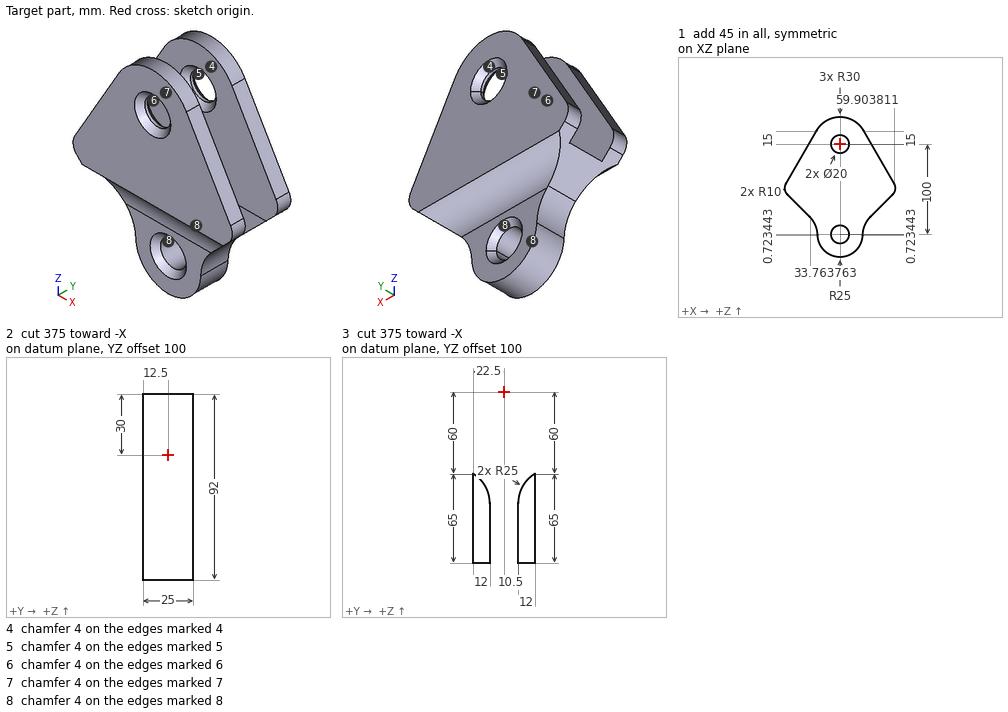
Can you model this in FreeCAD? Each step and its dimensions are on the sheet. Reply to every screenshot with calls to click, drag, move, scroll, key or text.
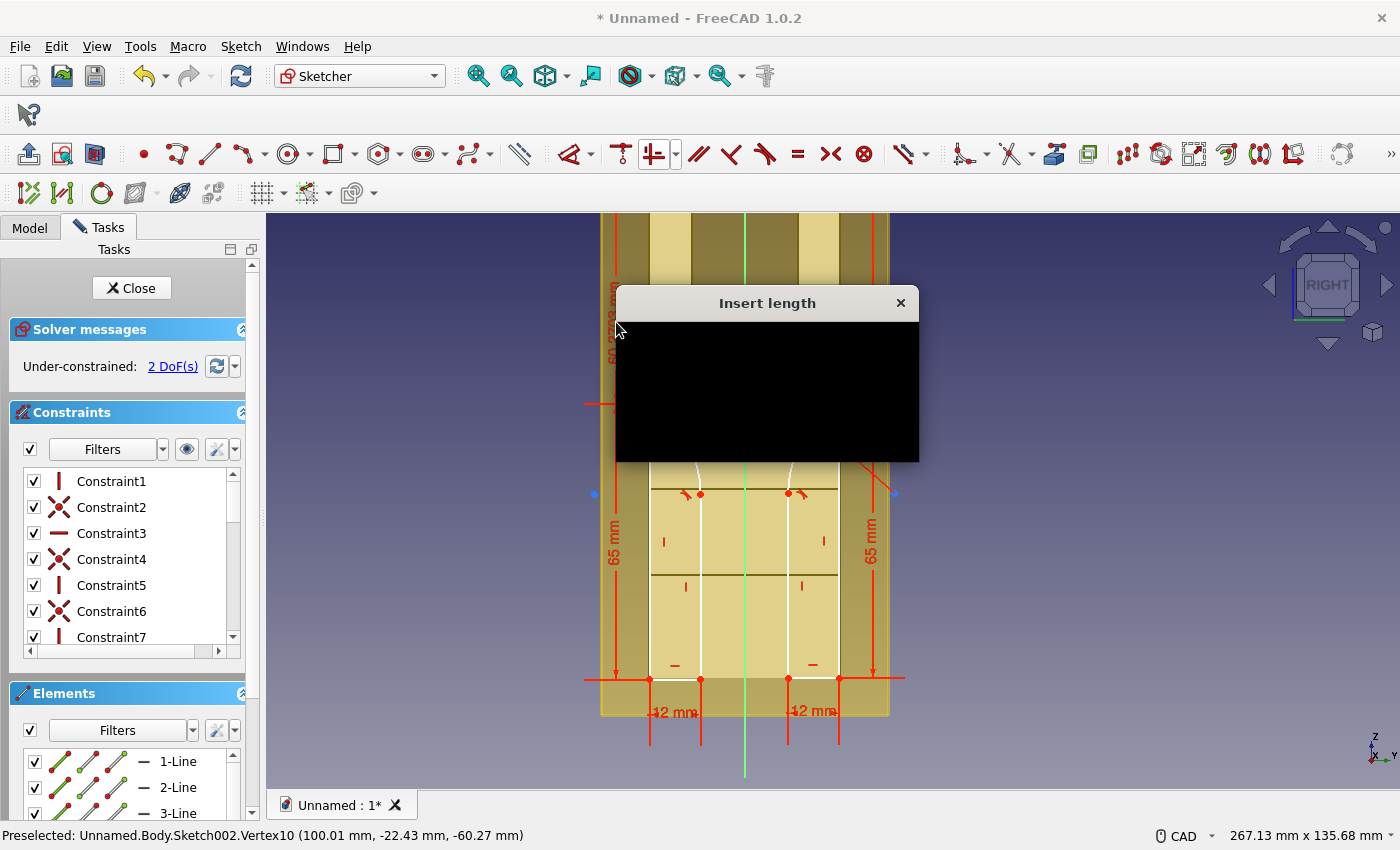
text(60)
key(Return)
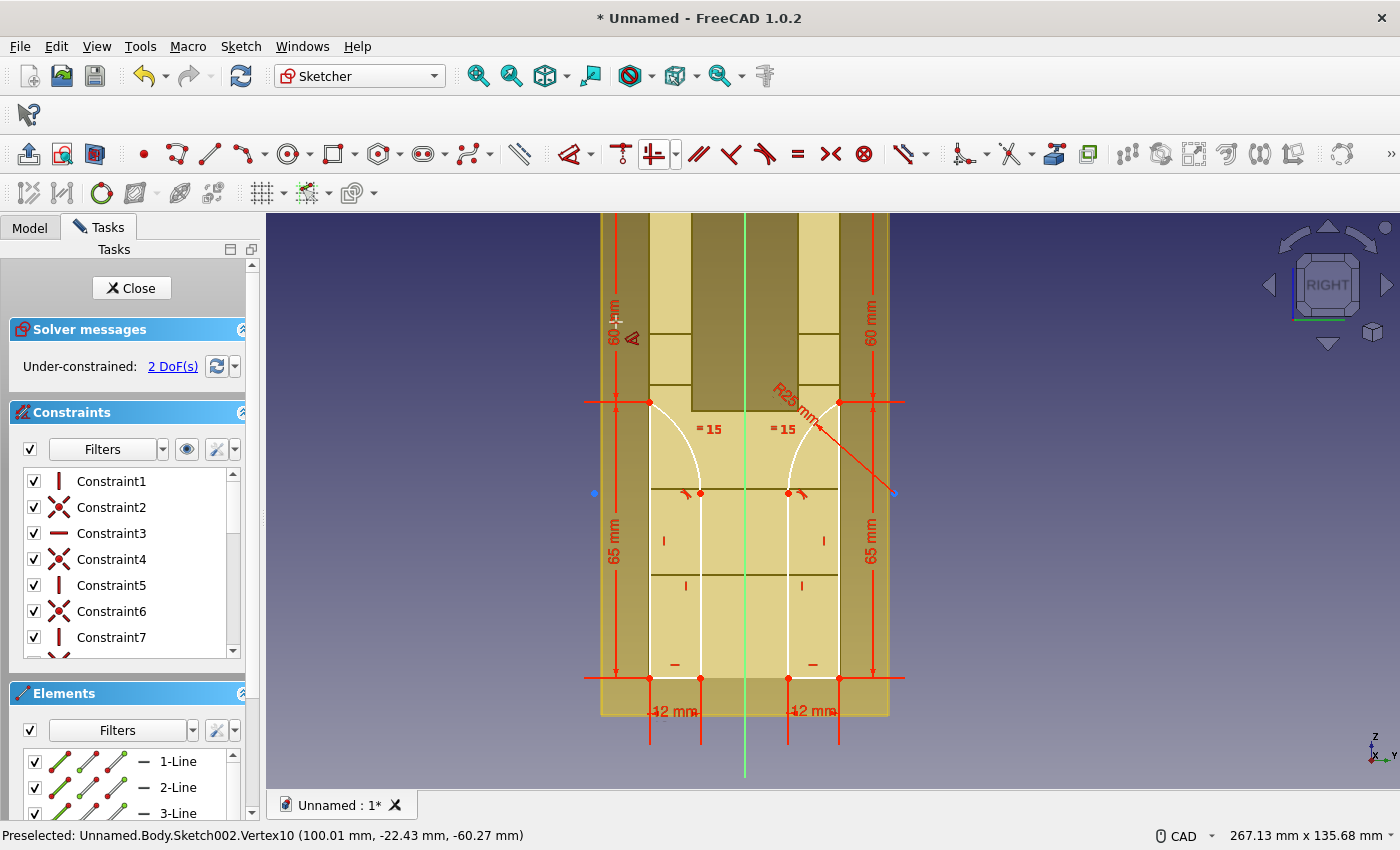
click(788, 493)
click(767, 527)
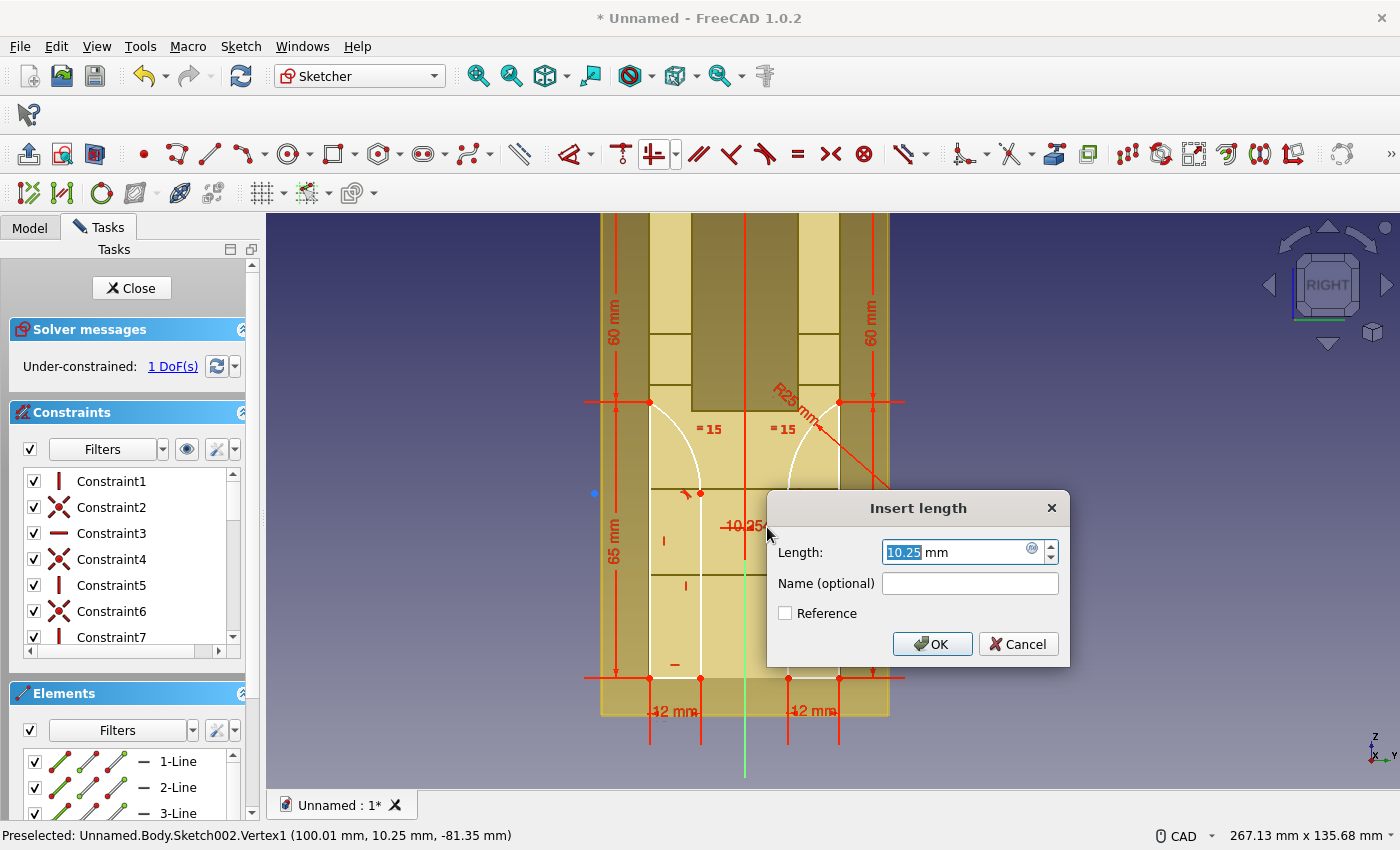
text(10.5)
key(Return)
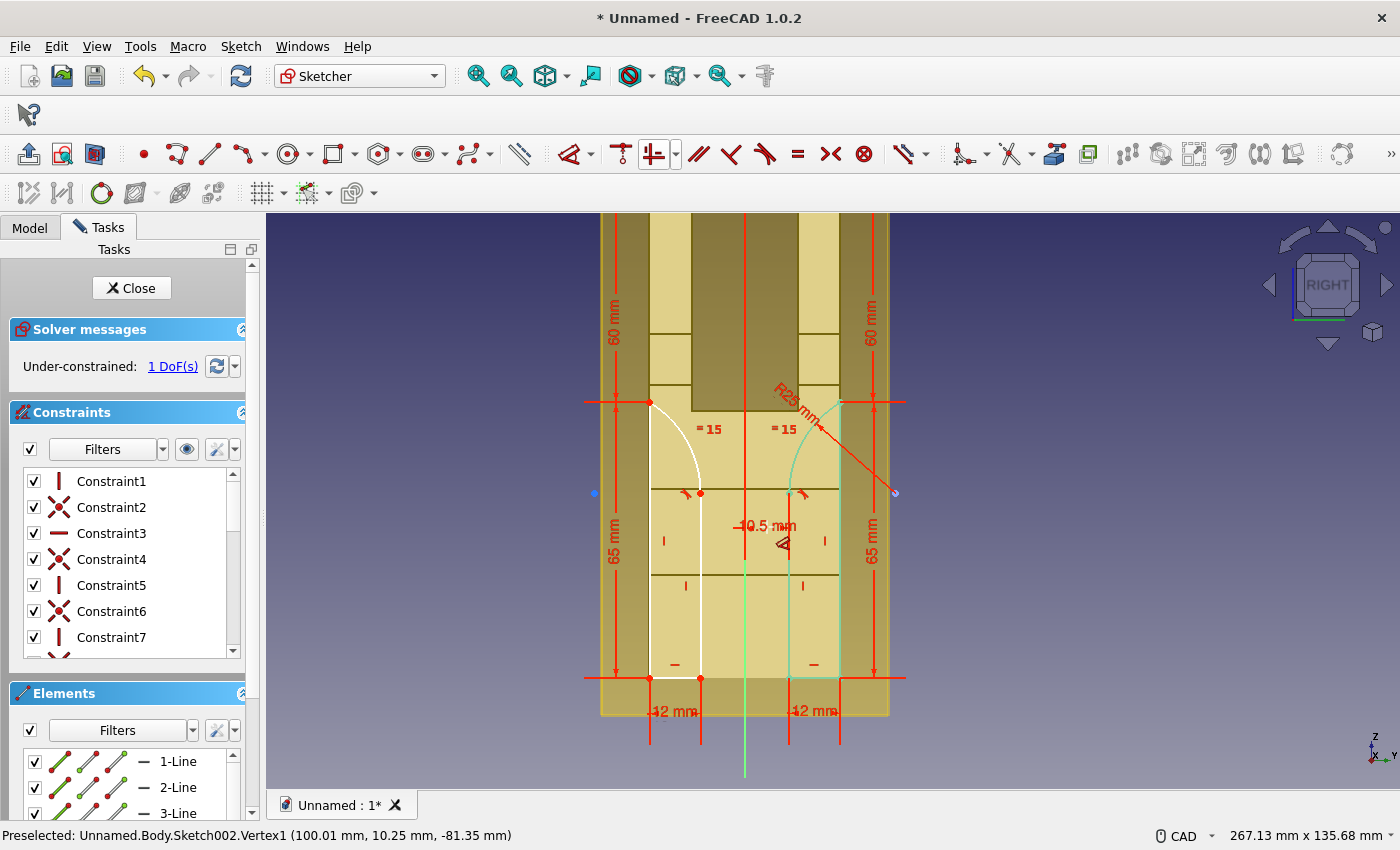
click(650, 402)
click(719, 436)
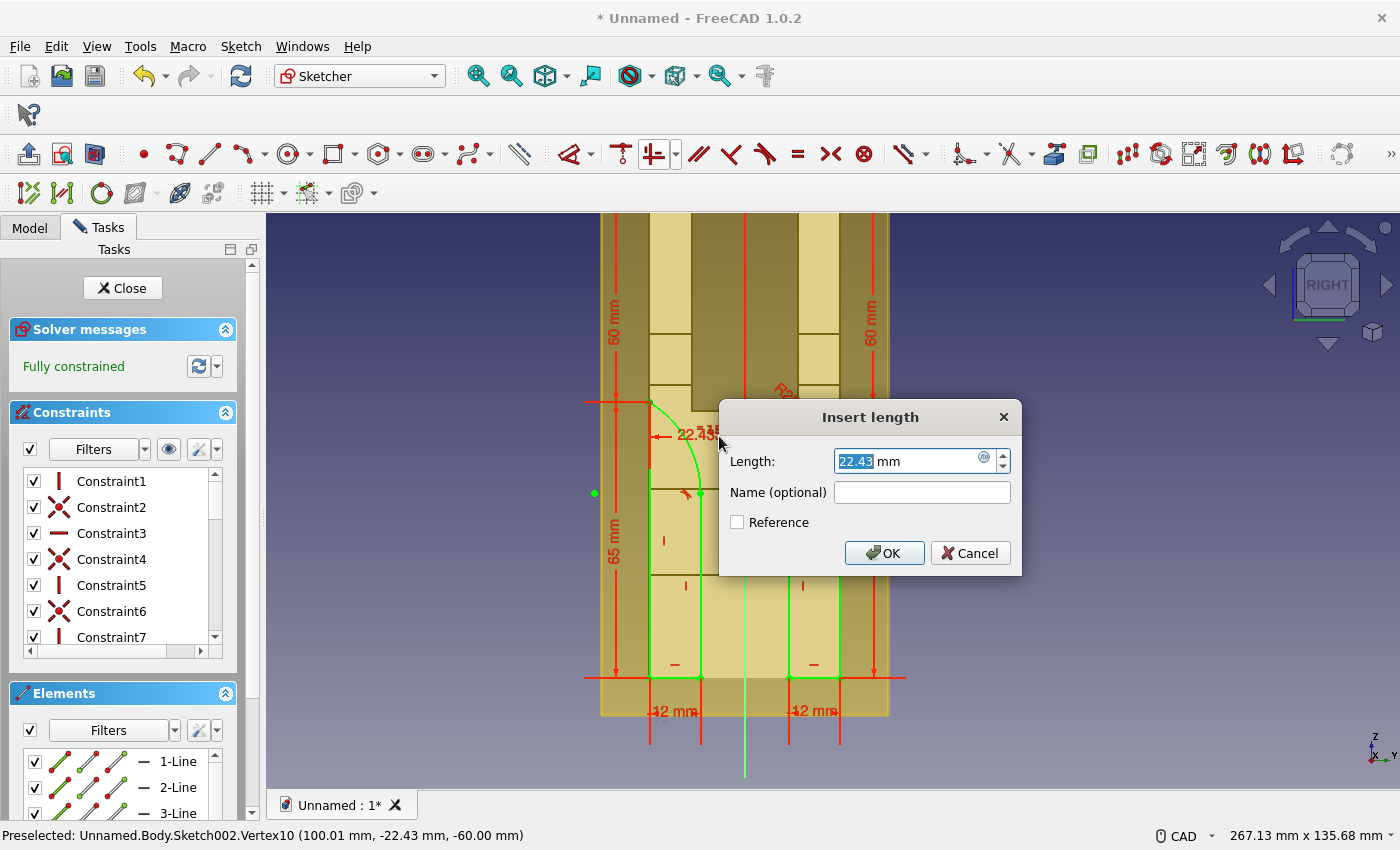
text(22.5)
key(Return)
key(Escape)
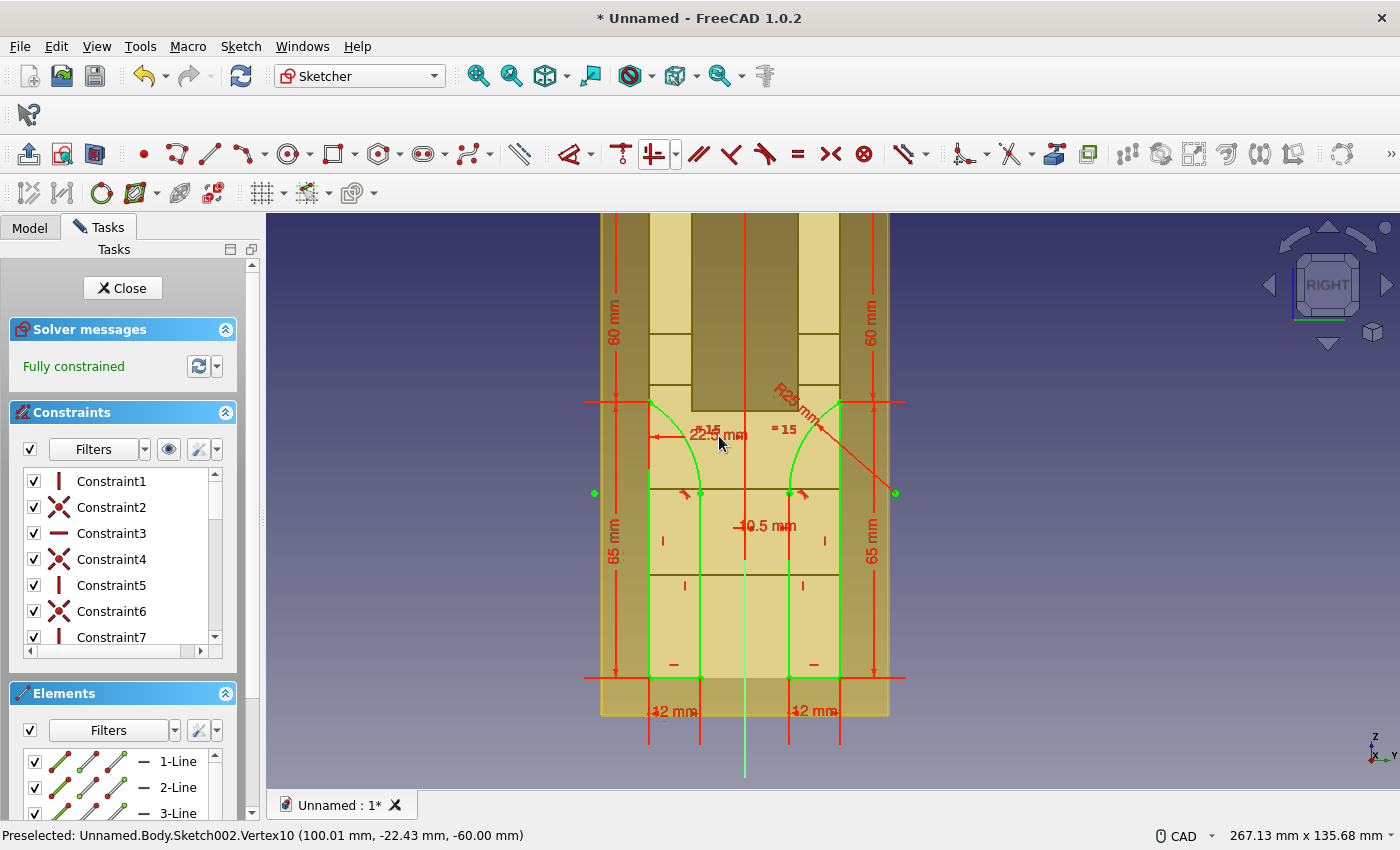
click(123, 288)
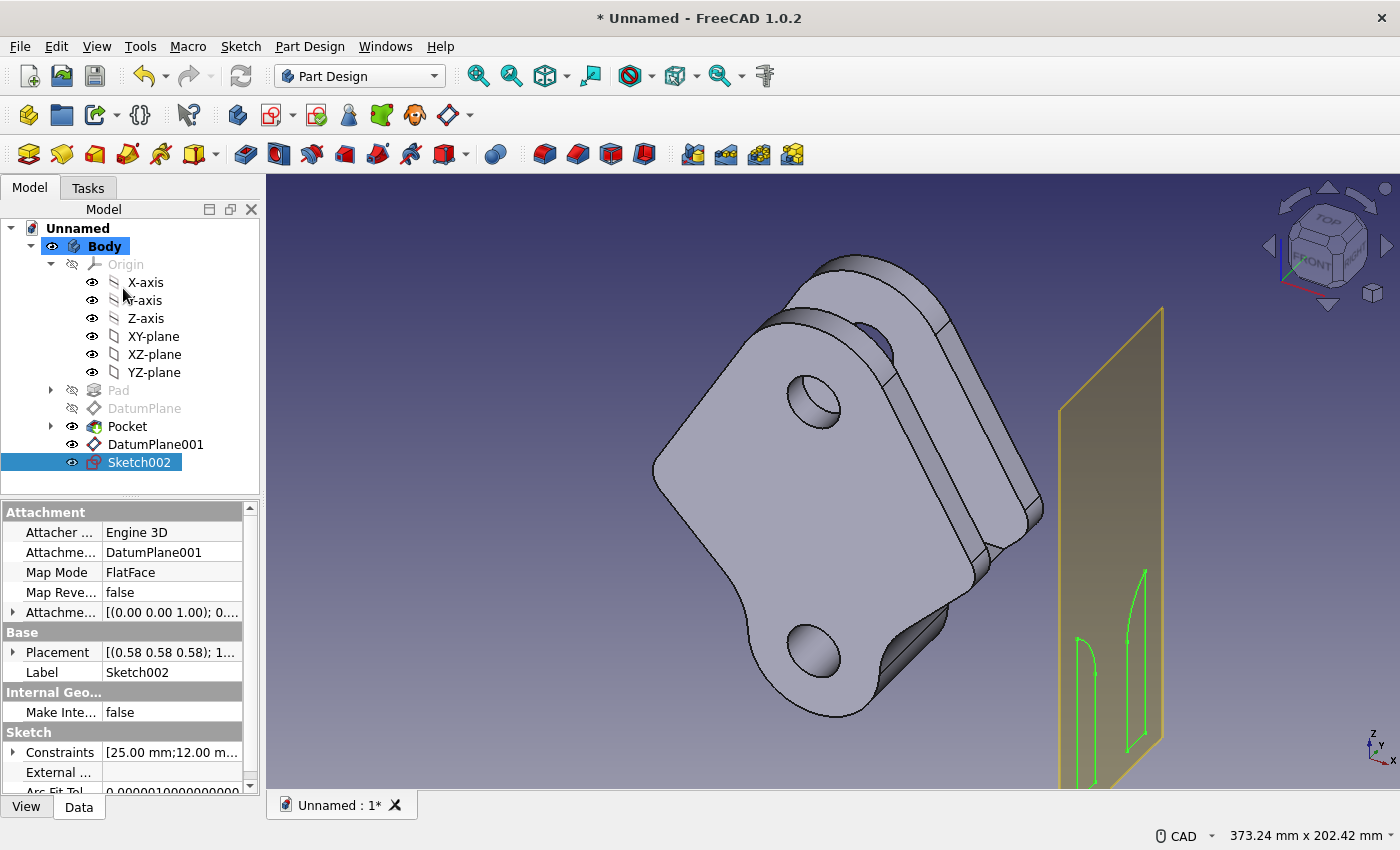
click(246, 154)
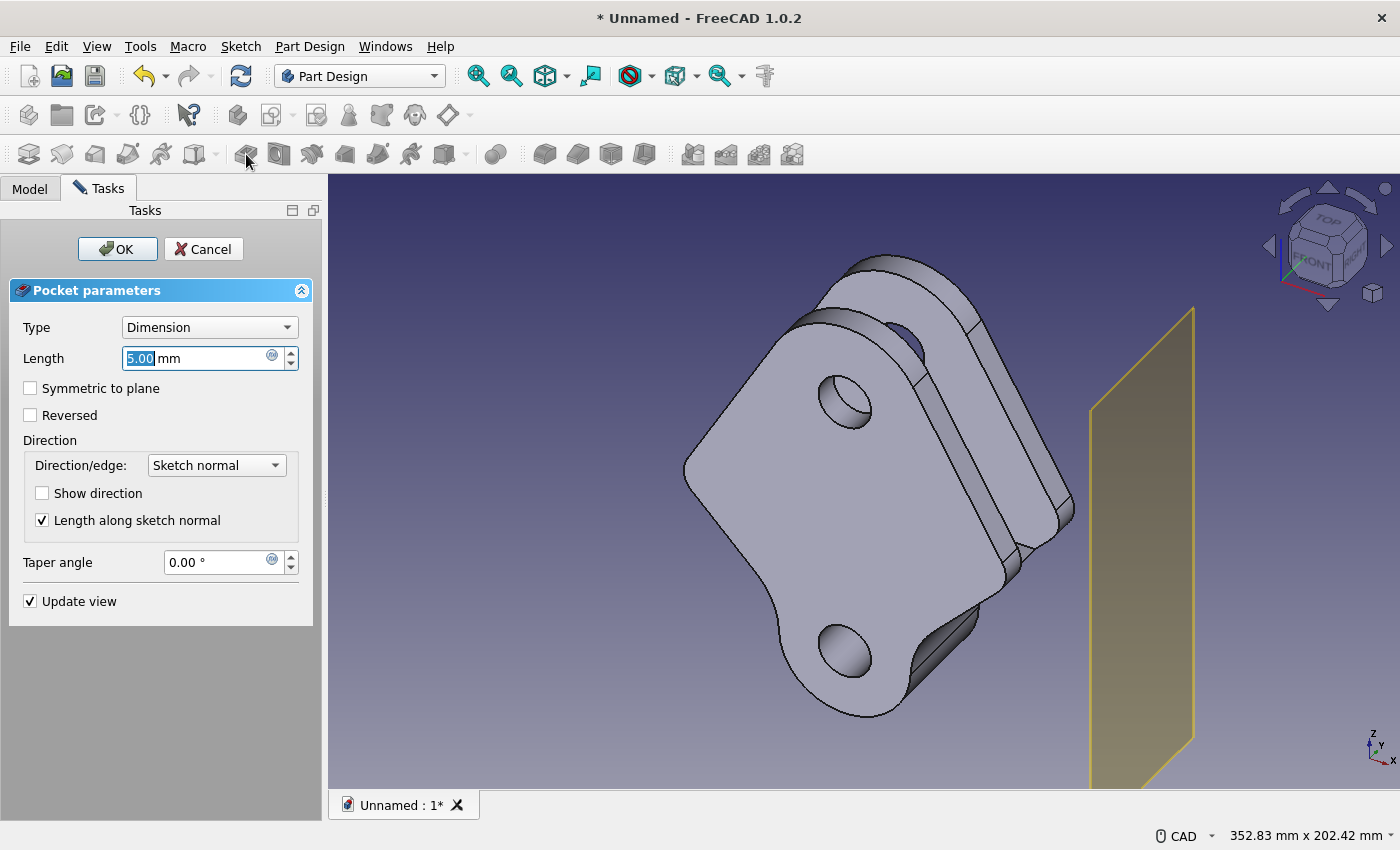
text(375)
key(Tab)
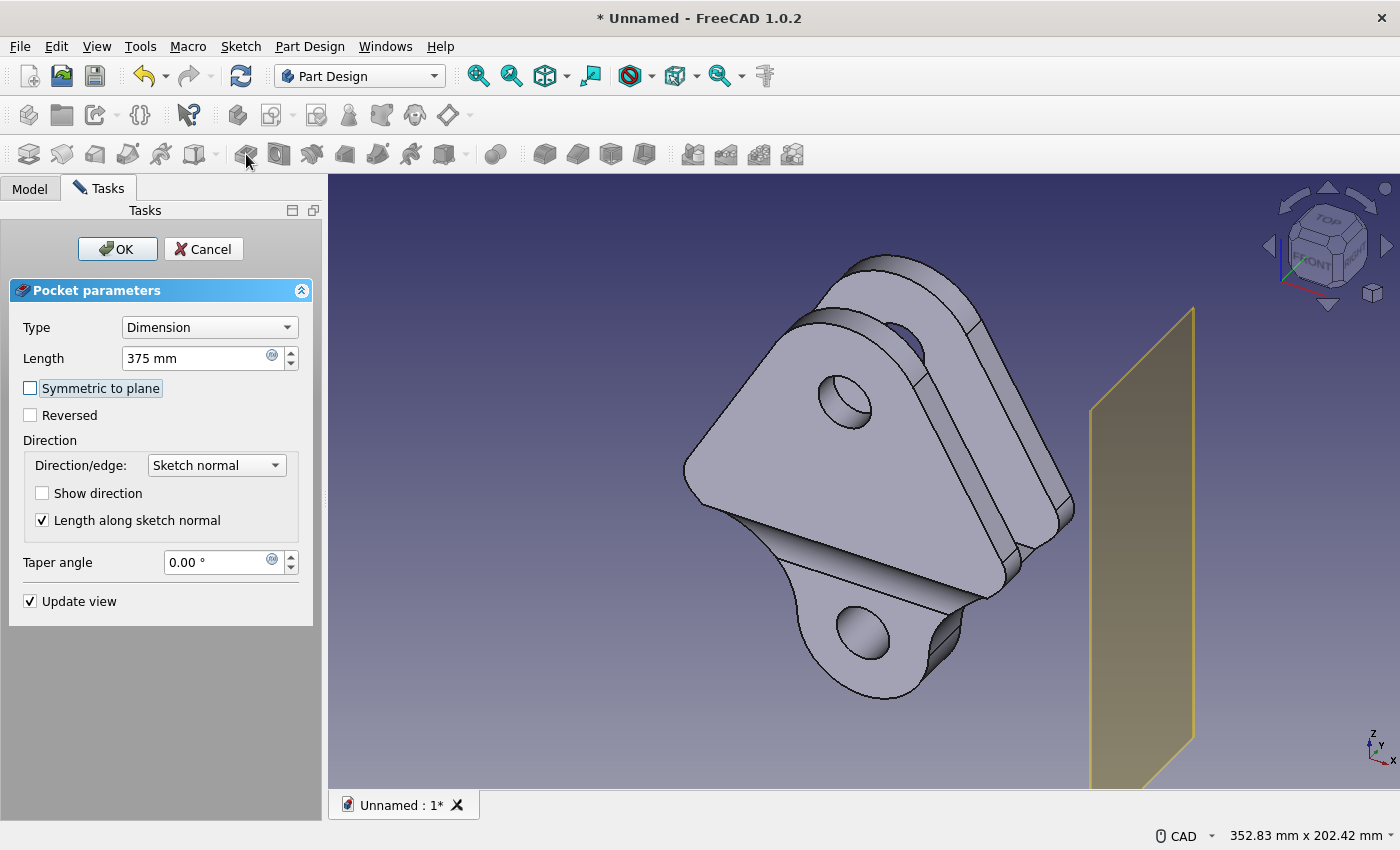
click(118, 249)